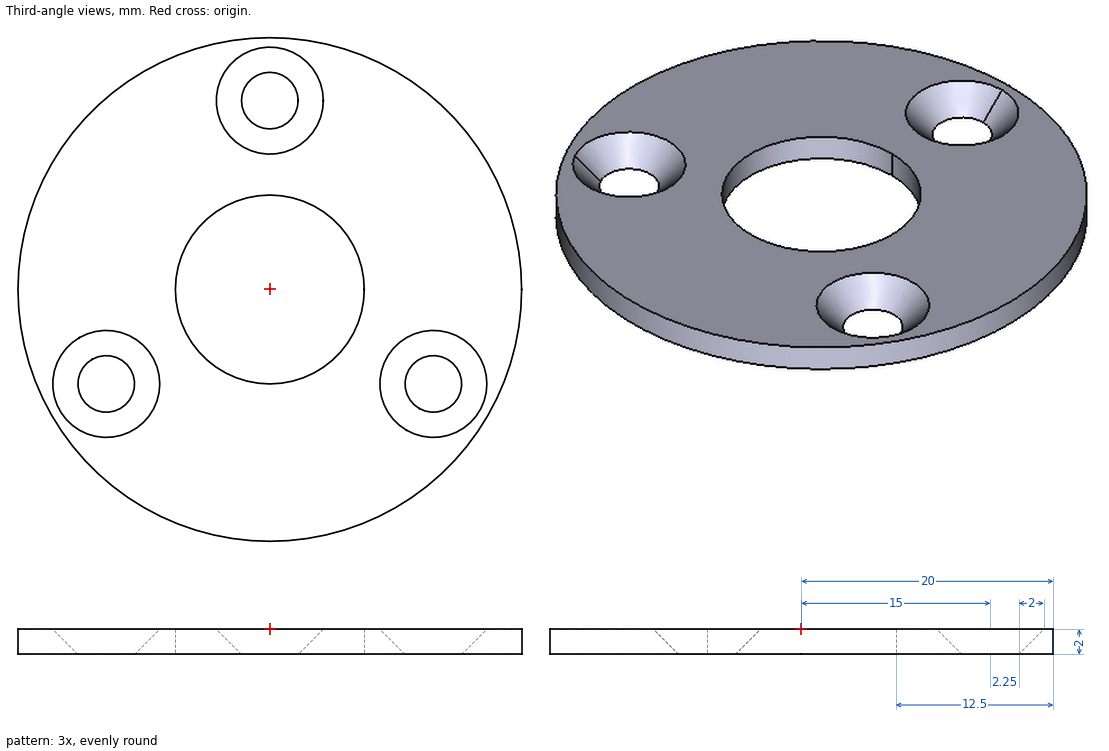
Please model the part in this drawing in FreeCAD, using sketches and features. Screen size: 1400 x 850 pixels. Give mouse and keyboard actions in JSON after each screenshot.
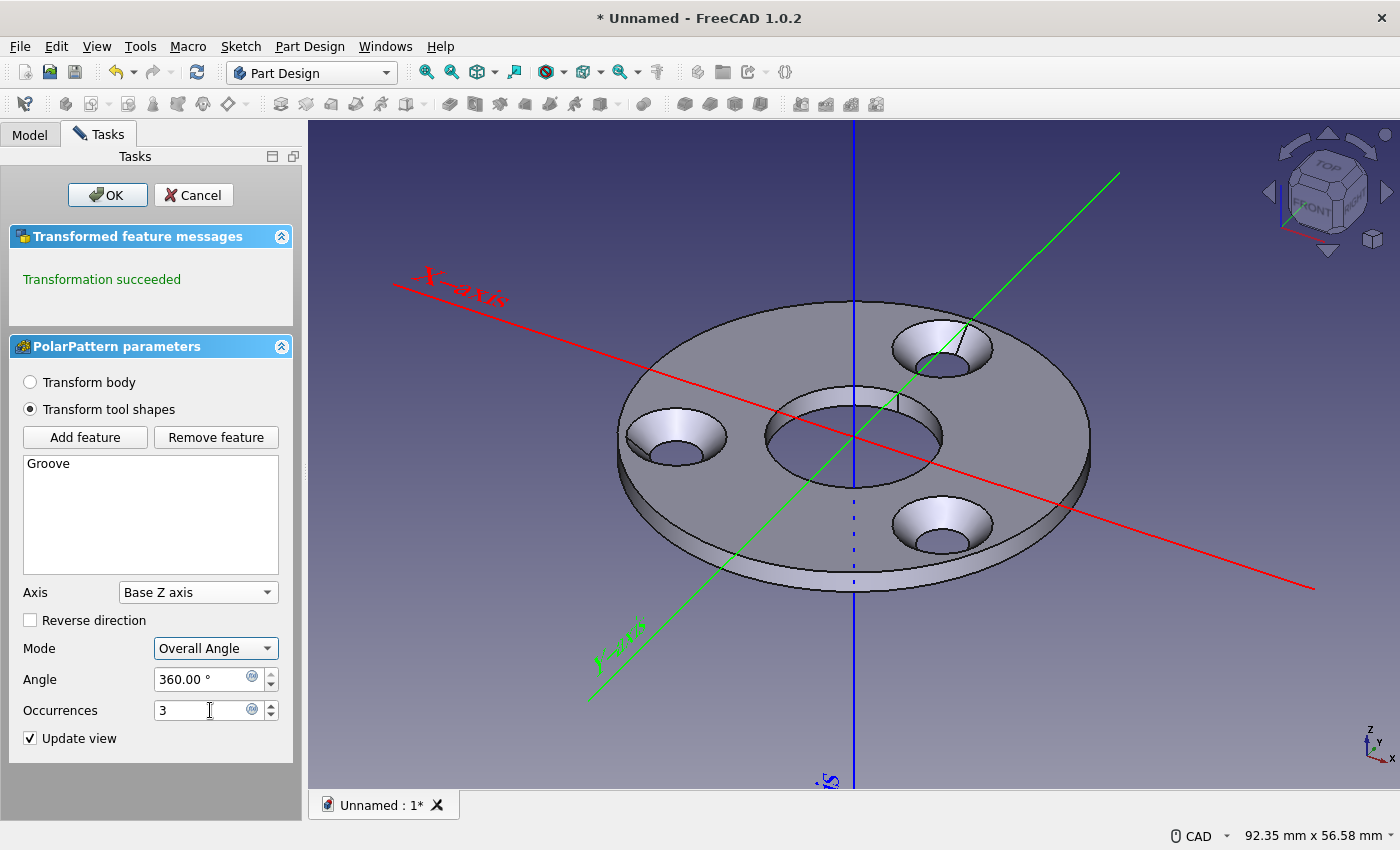
{"action": "left_click", "coordinate": [108, 195]}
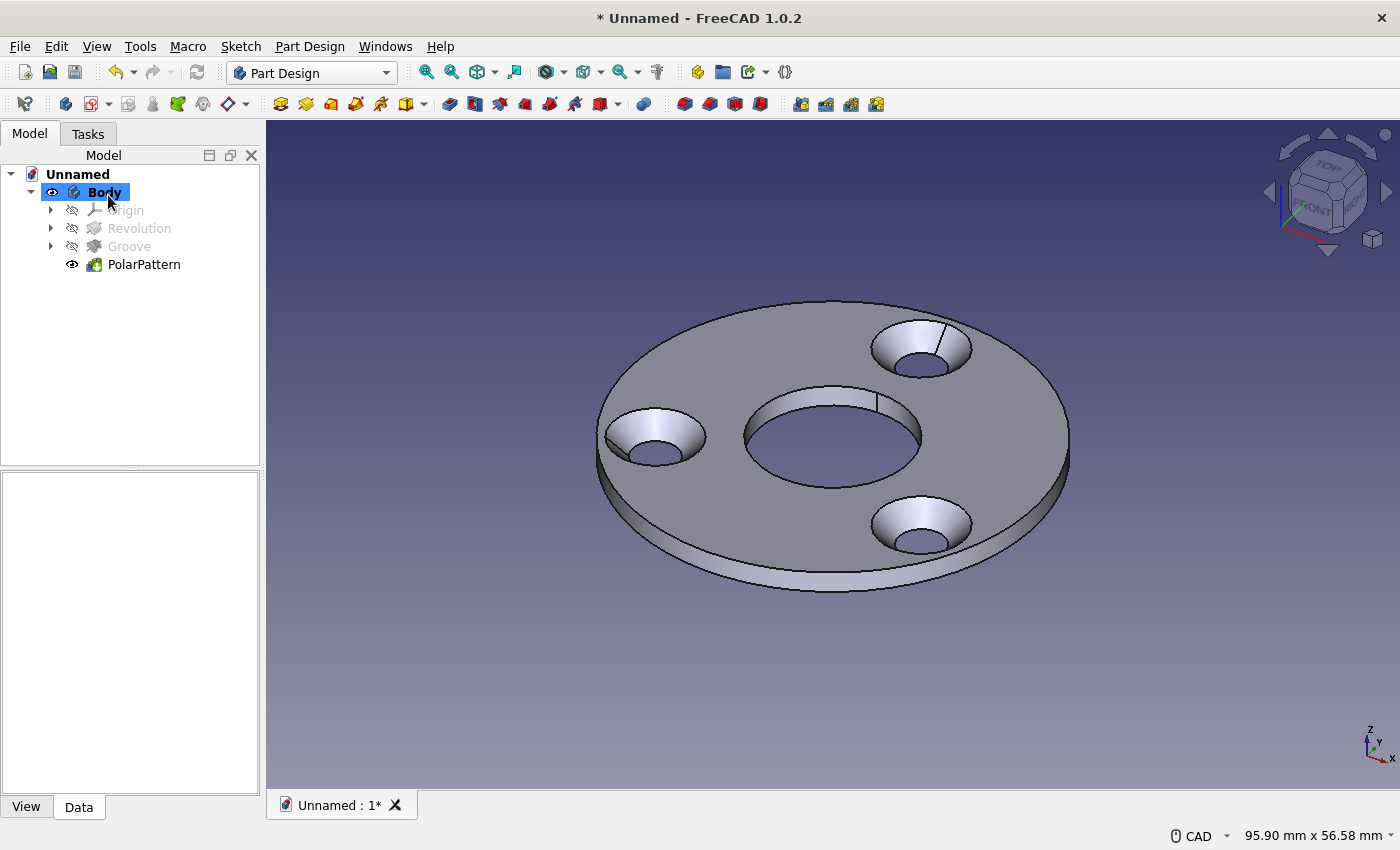
{"action": "key", "text": "0"}